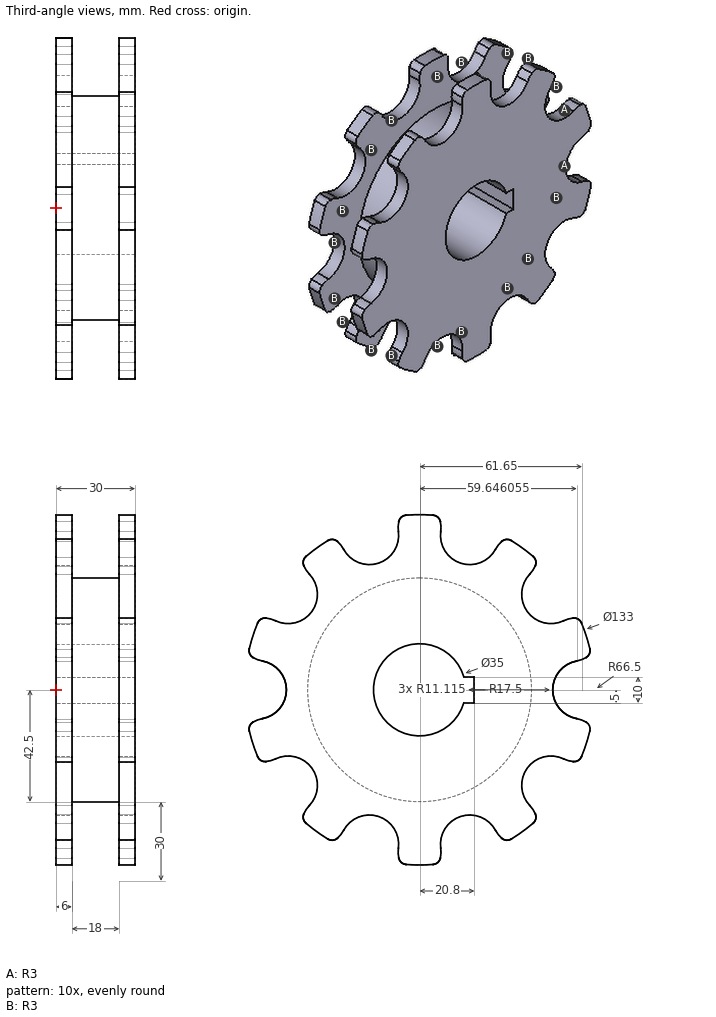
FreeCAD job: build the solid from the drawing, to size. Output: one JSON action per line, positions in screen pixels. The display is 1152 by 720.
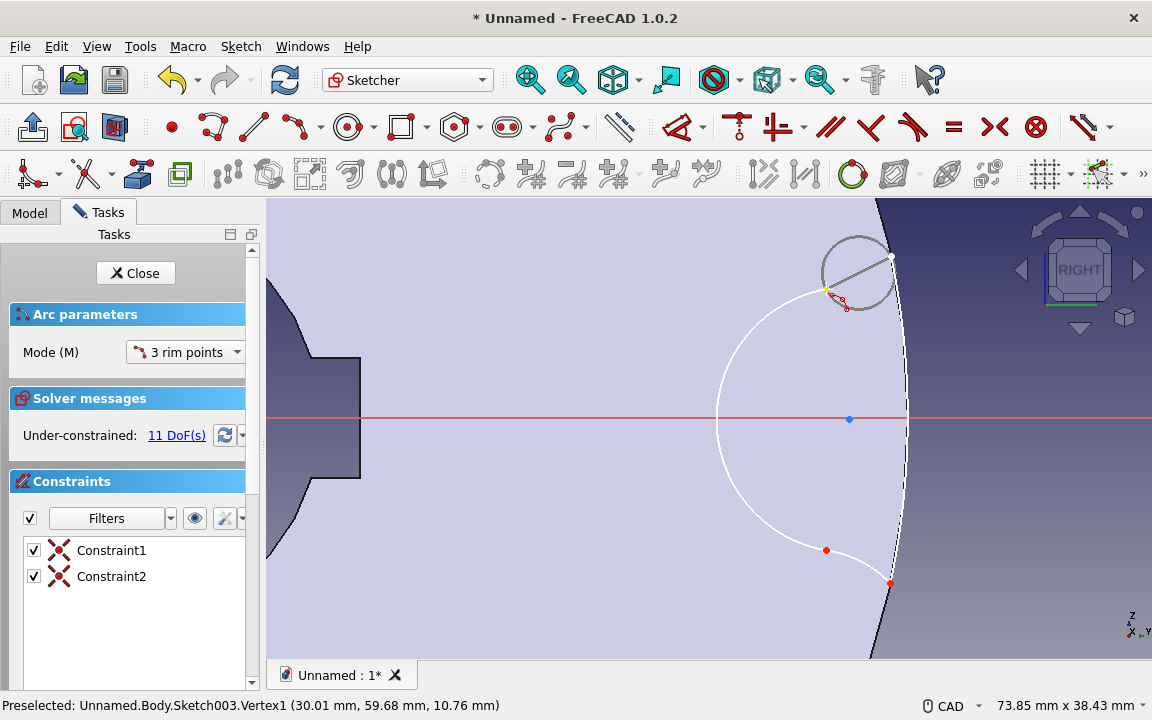
{"action": "scroll", "coordinate": [861, 276], "scroll_direction": "up", "scroll_amount": 6}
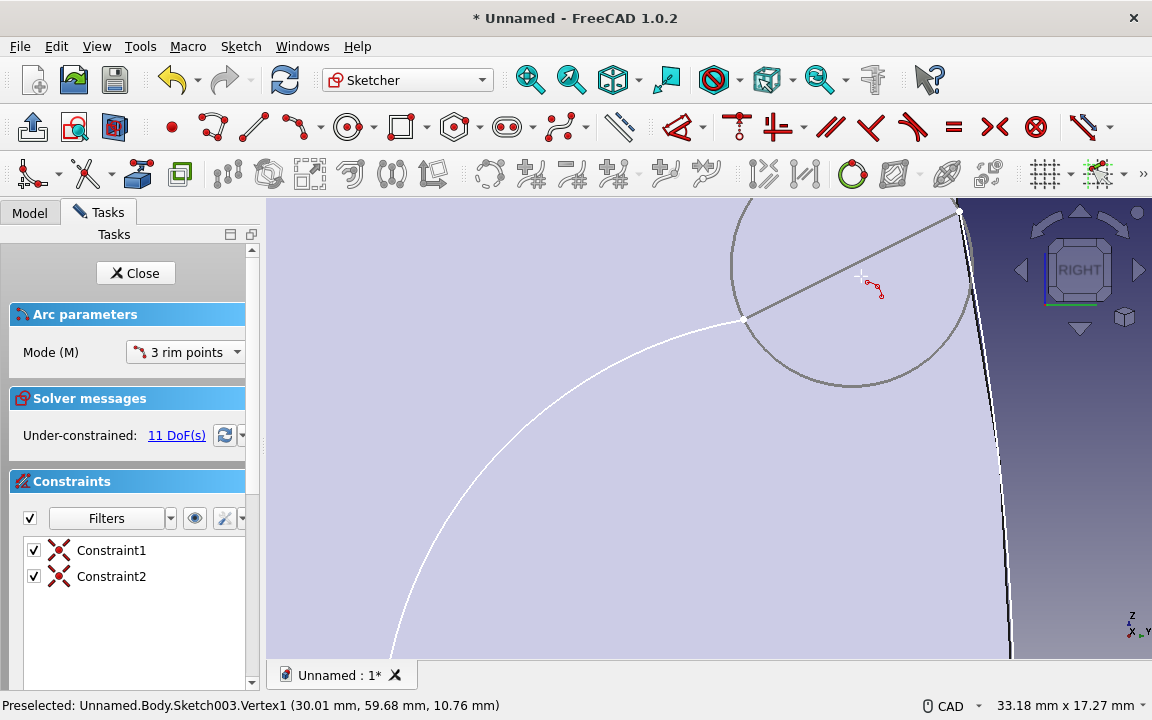
{"action": "left_click", "coordinate": [858, 274]}
{"action": "key", "text": "Escape"}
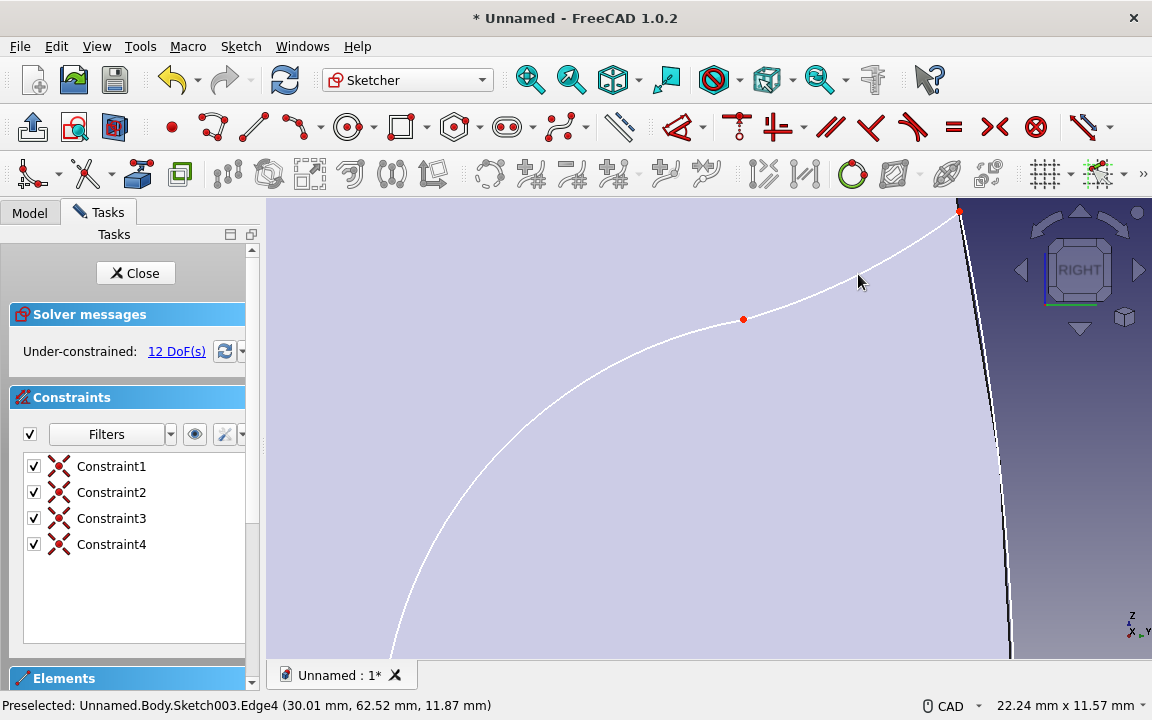
{"action": "scroll", "coordinate": [881, 348], "scroll_direction": "down", "scroll_amount": 8}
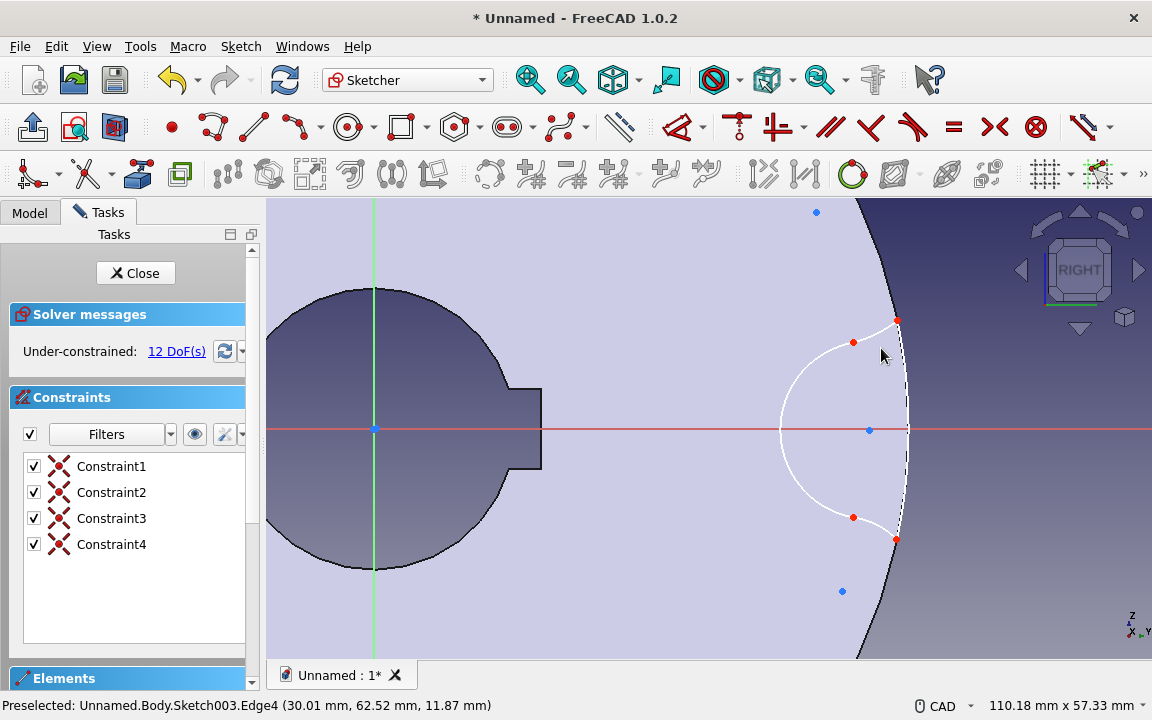
{"action": "left_click", "coordinate": [794, 383]}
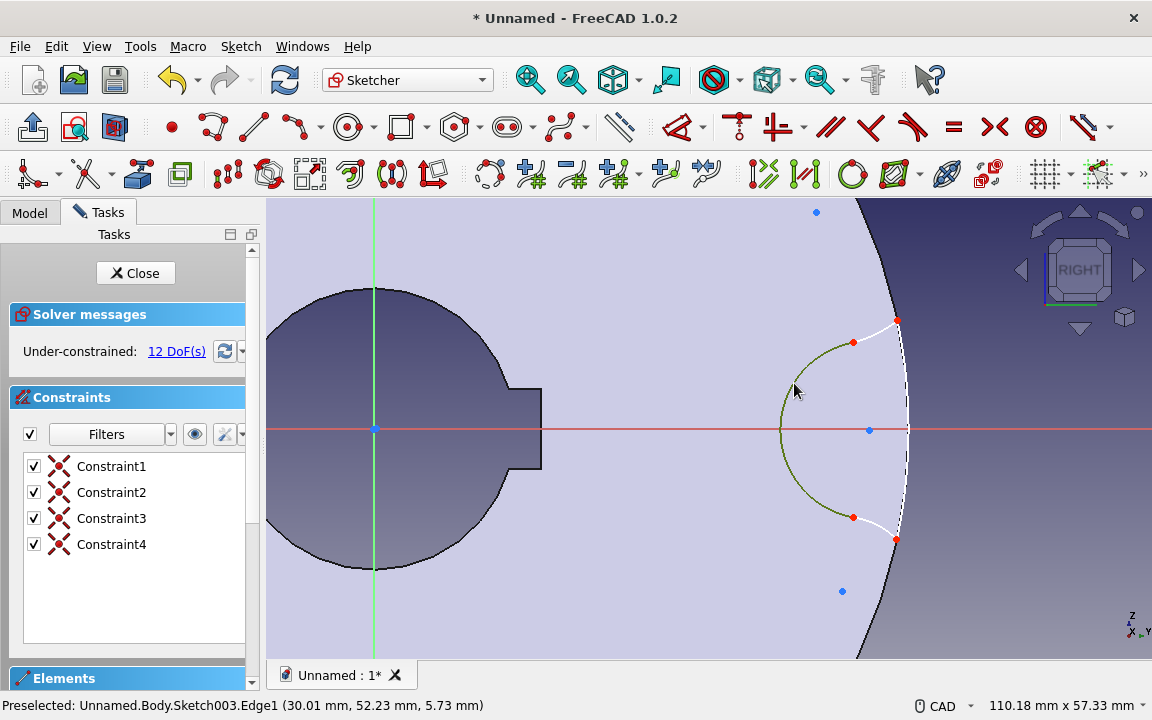
{"action": "left_click", "coordinate": [886, 530]}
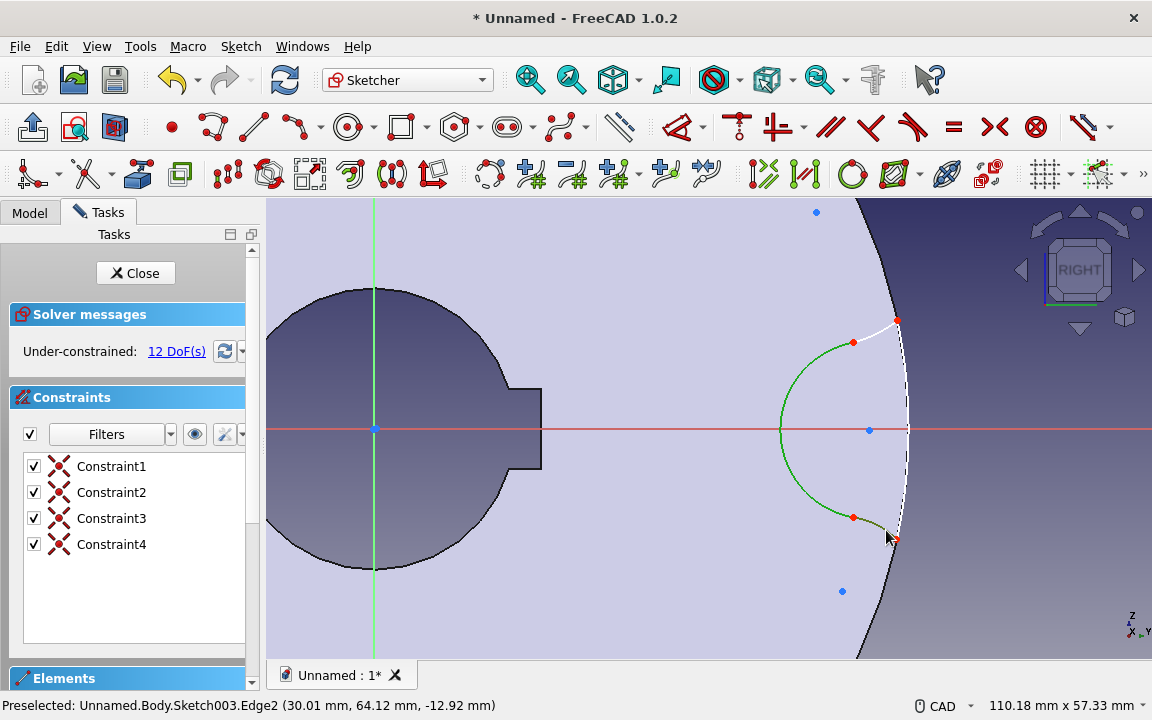
{"action": "left_click", "coordinate": [913, 128]}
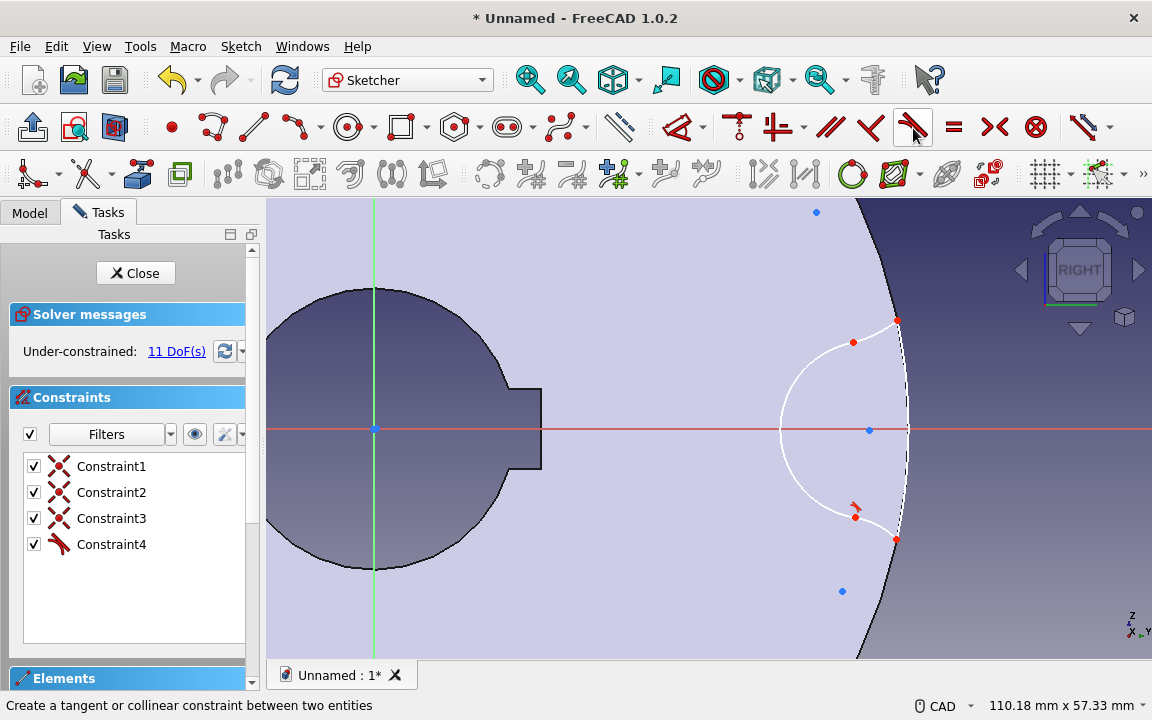
{"action": "left_click", "coordinate": [794, 383]}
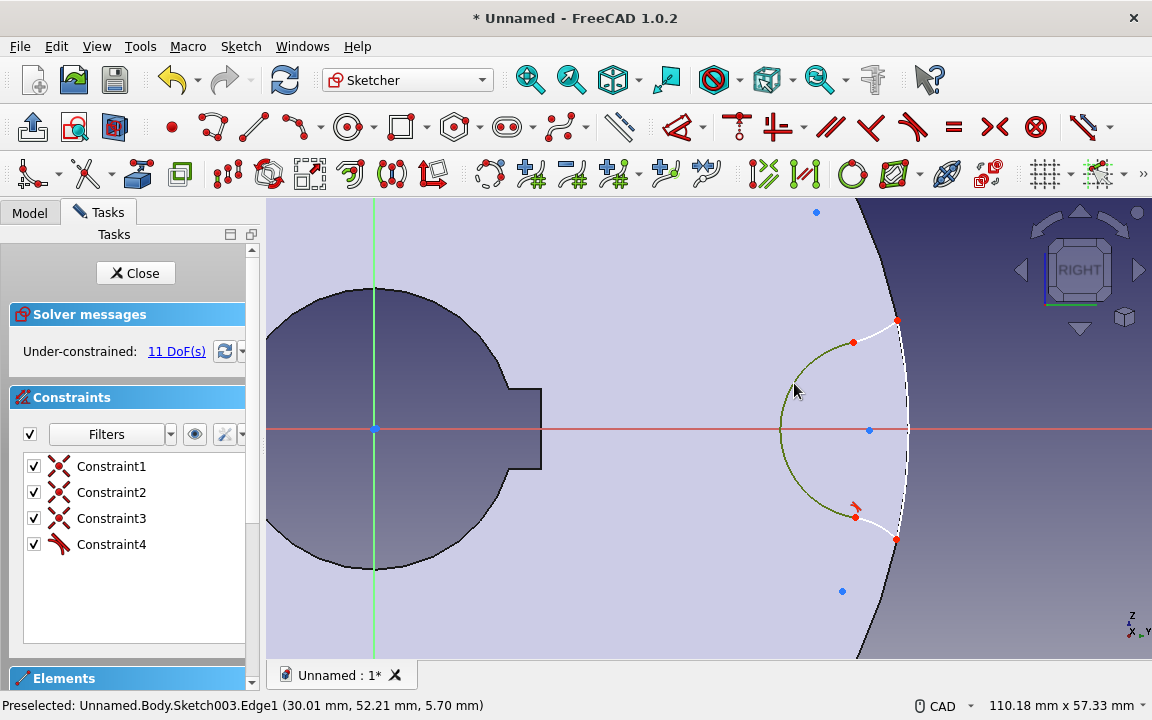
{"action": "left_click", "coordinate": [868, 338]}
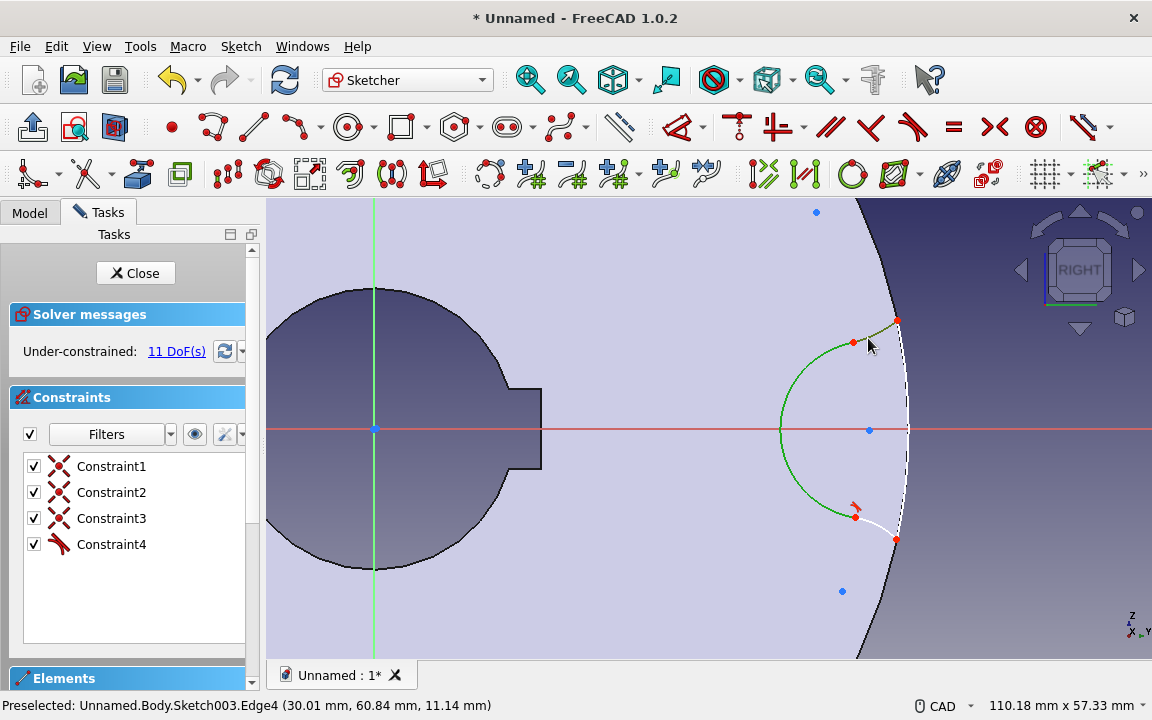
{"action": "left_click", "coordinate": [913, 128]}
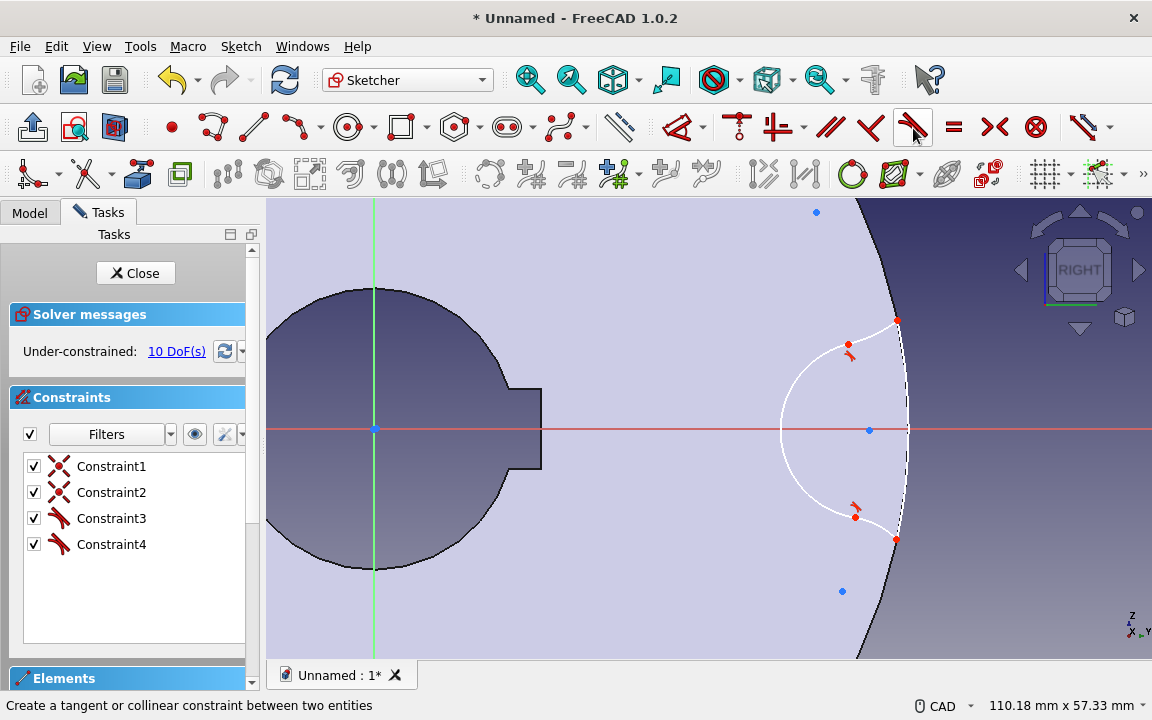
{"action": "left_click_drag", "start_coordinate": [364, 419], "coordinate": [386, 439]}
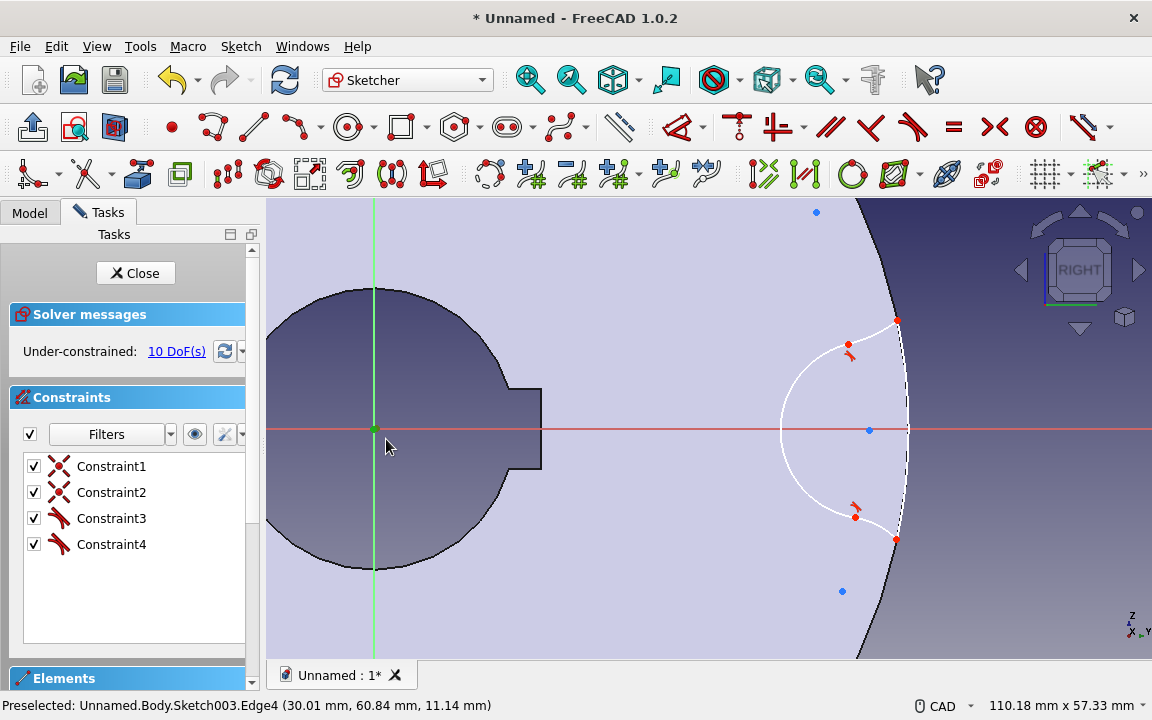
{"action": "left_click", "coordinate": [737, 128]}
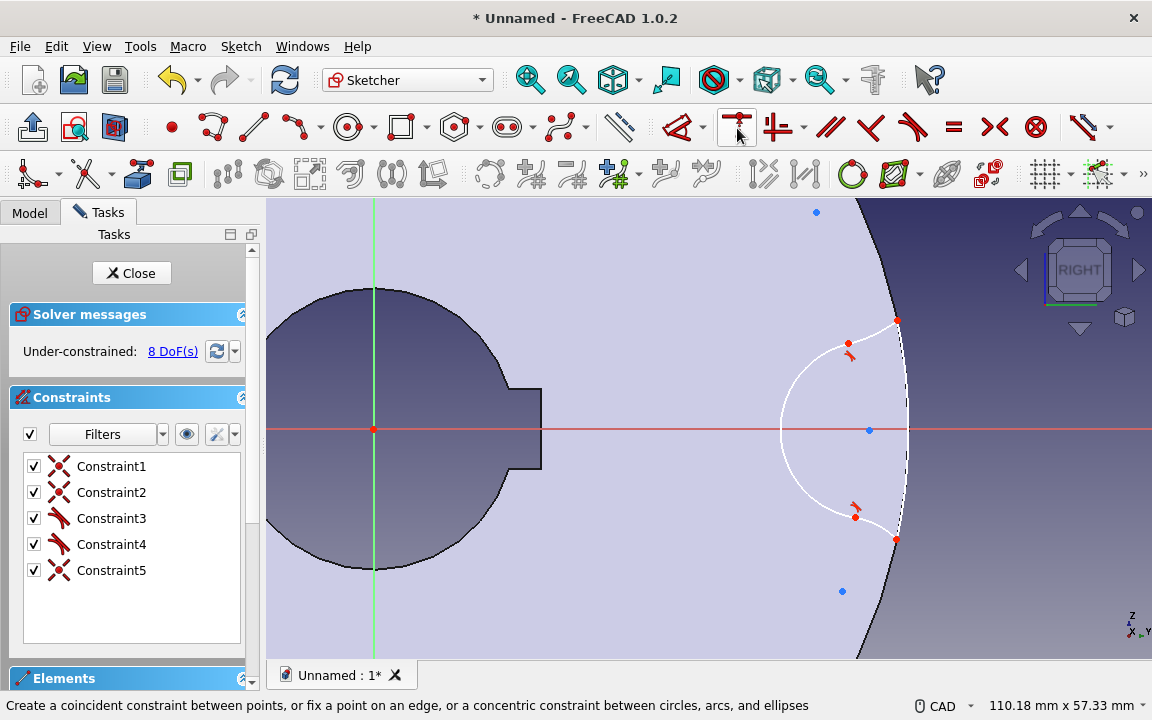
{"action": "left_click", "coordinate": [792, 387]}